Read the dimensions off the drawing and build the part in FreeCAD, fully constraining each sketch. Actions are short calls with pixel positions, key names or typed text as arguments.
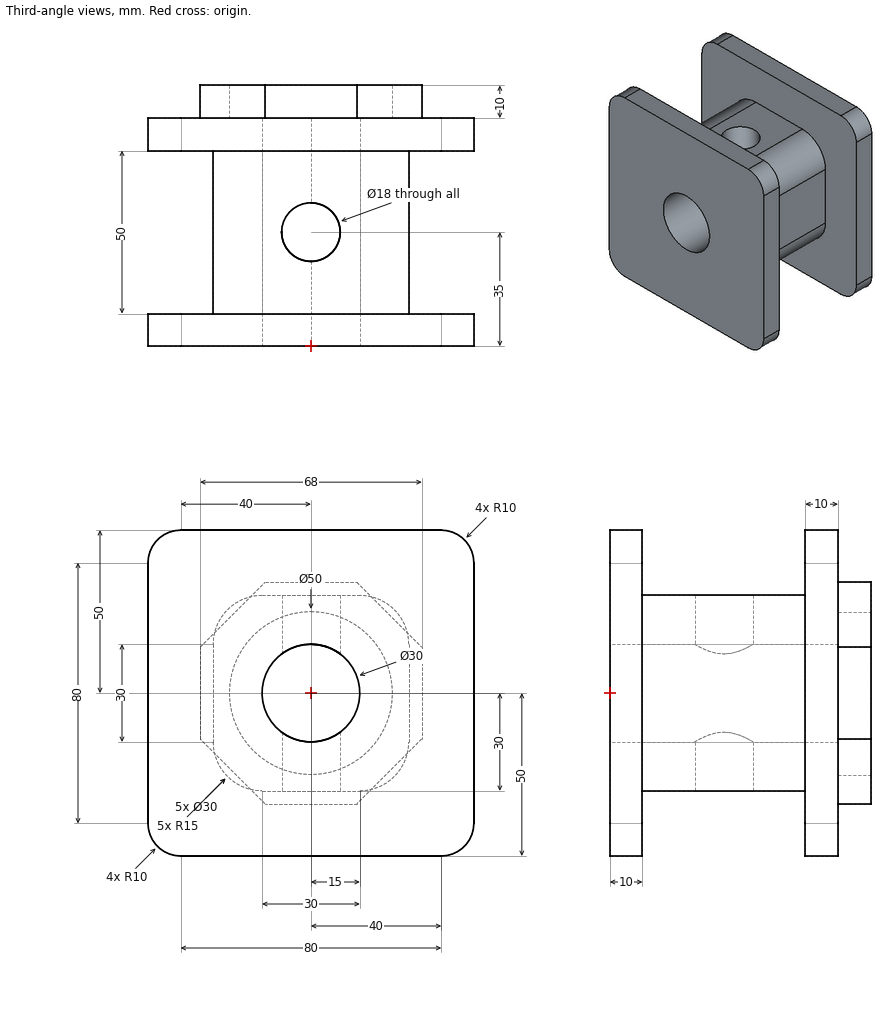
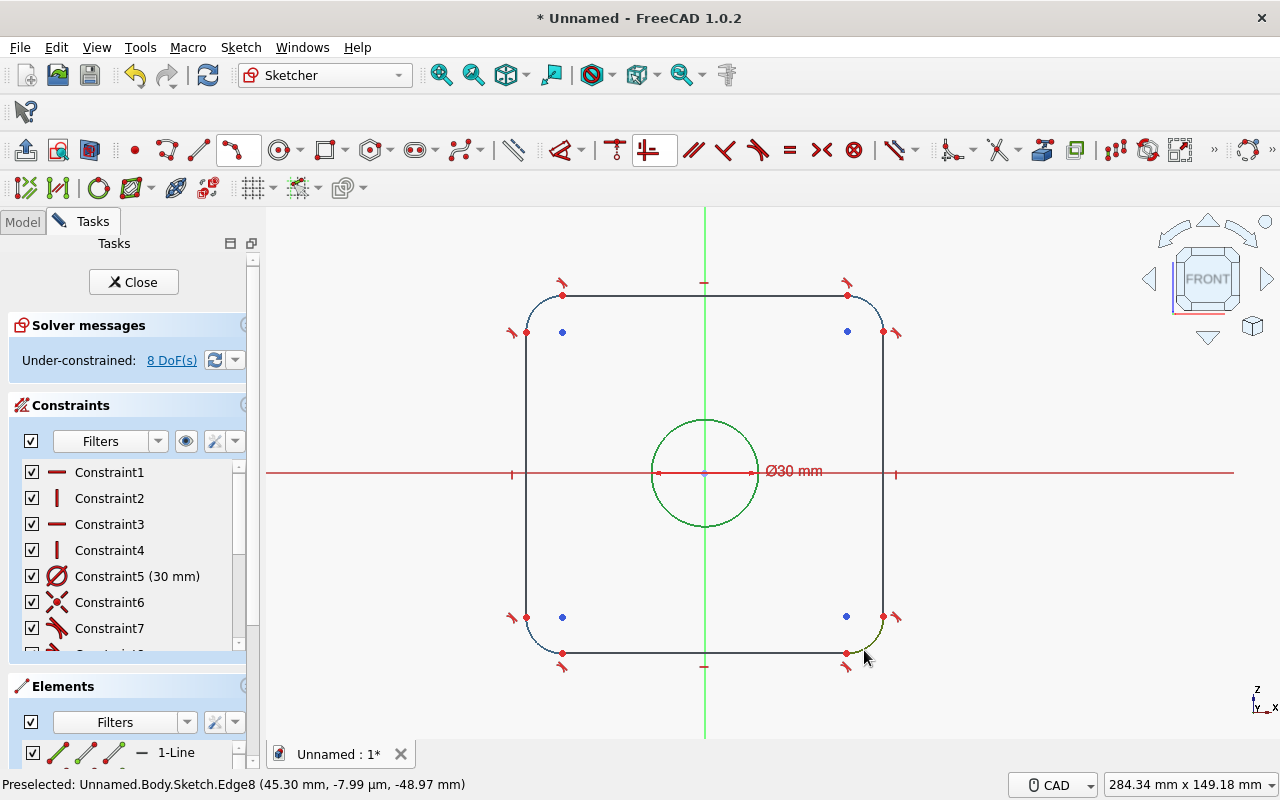
click(790, 150)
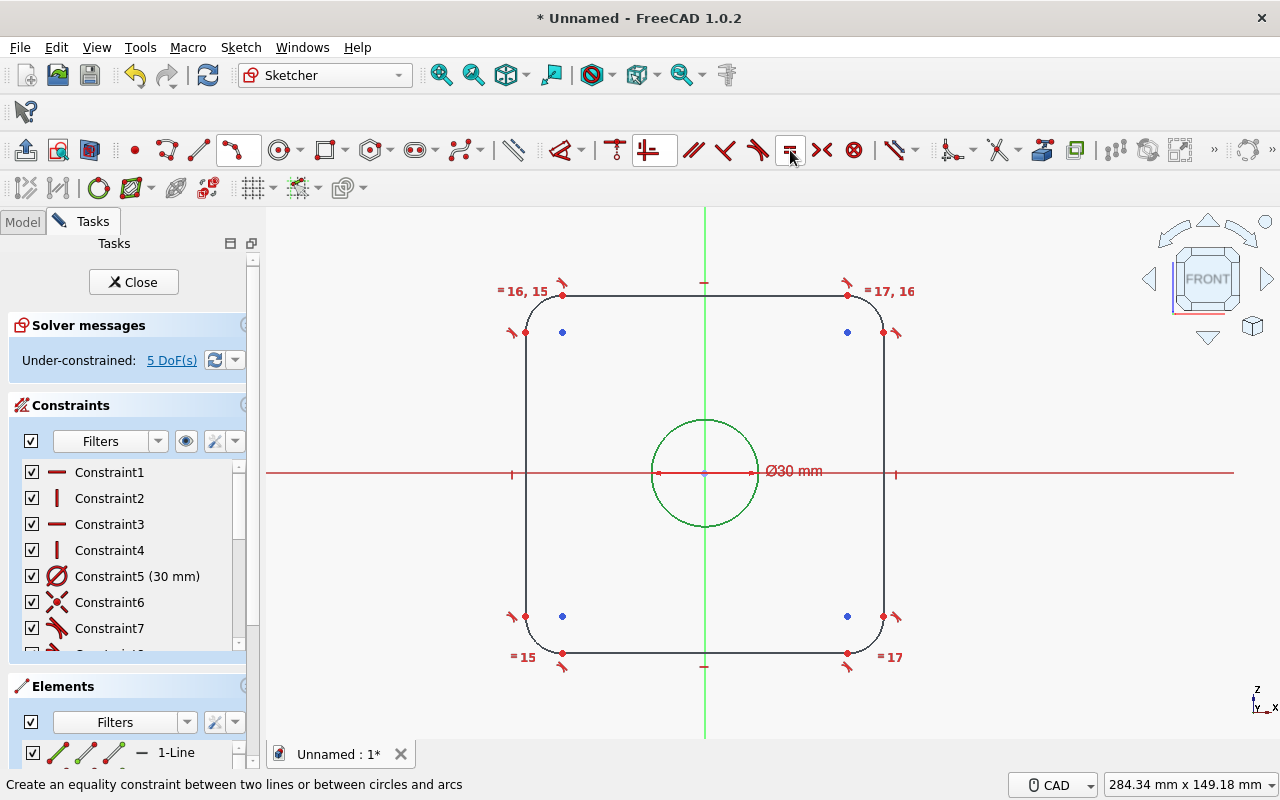
click(560, 150)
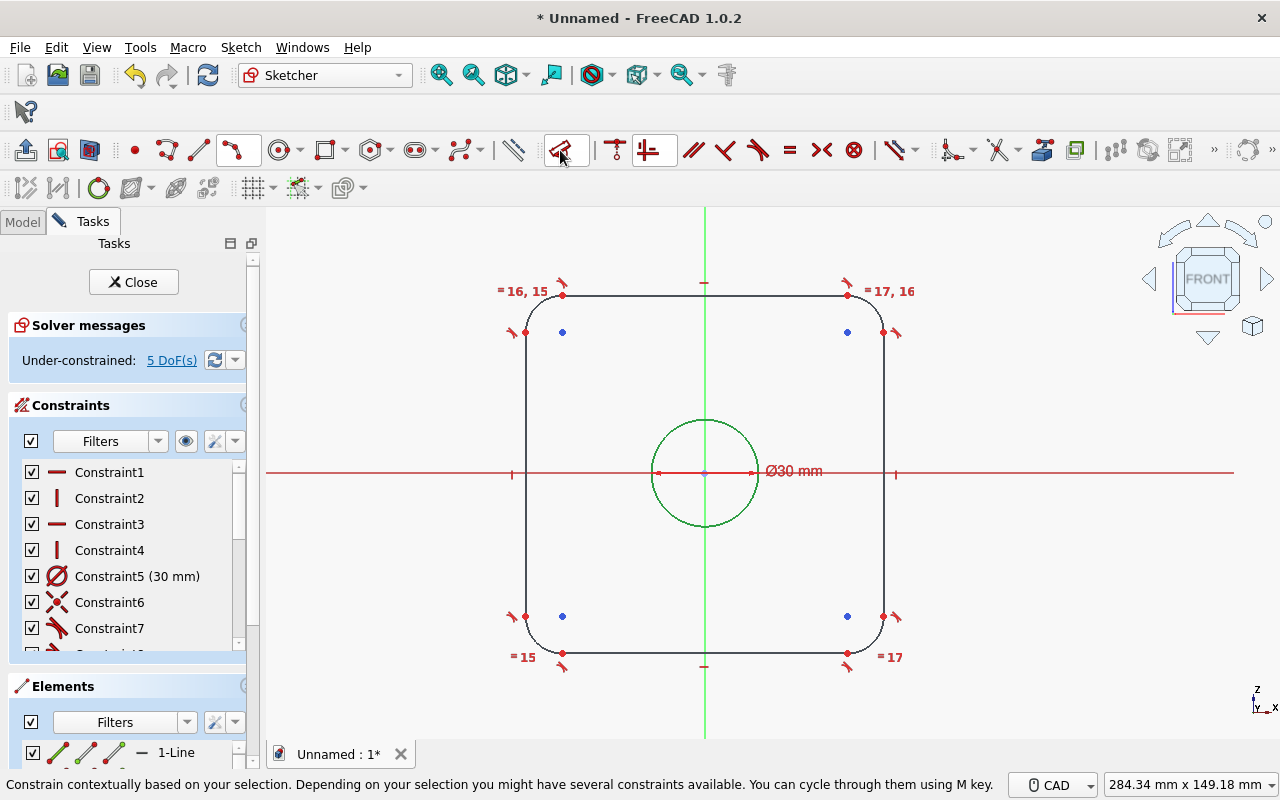
click(530, 634)
click(502, 649)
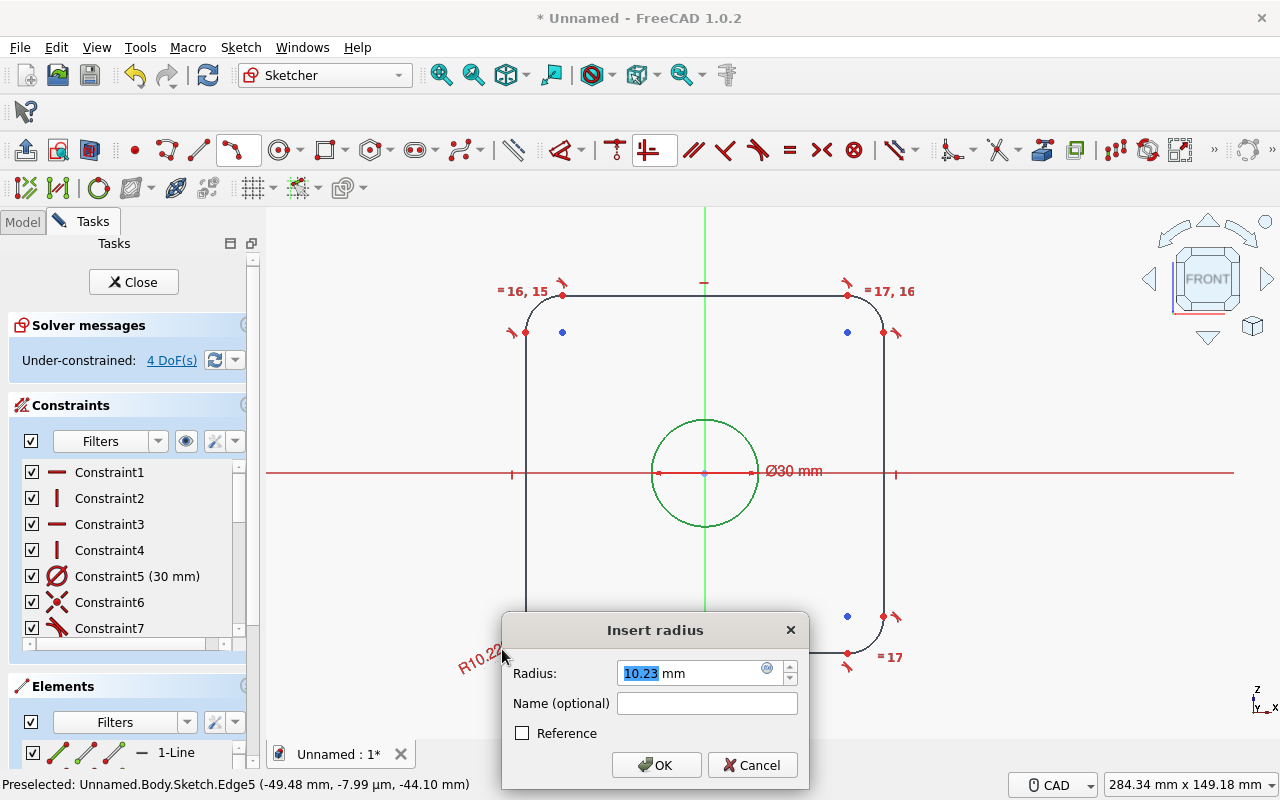
text(10)
key(Return)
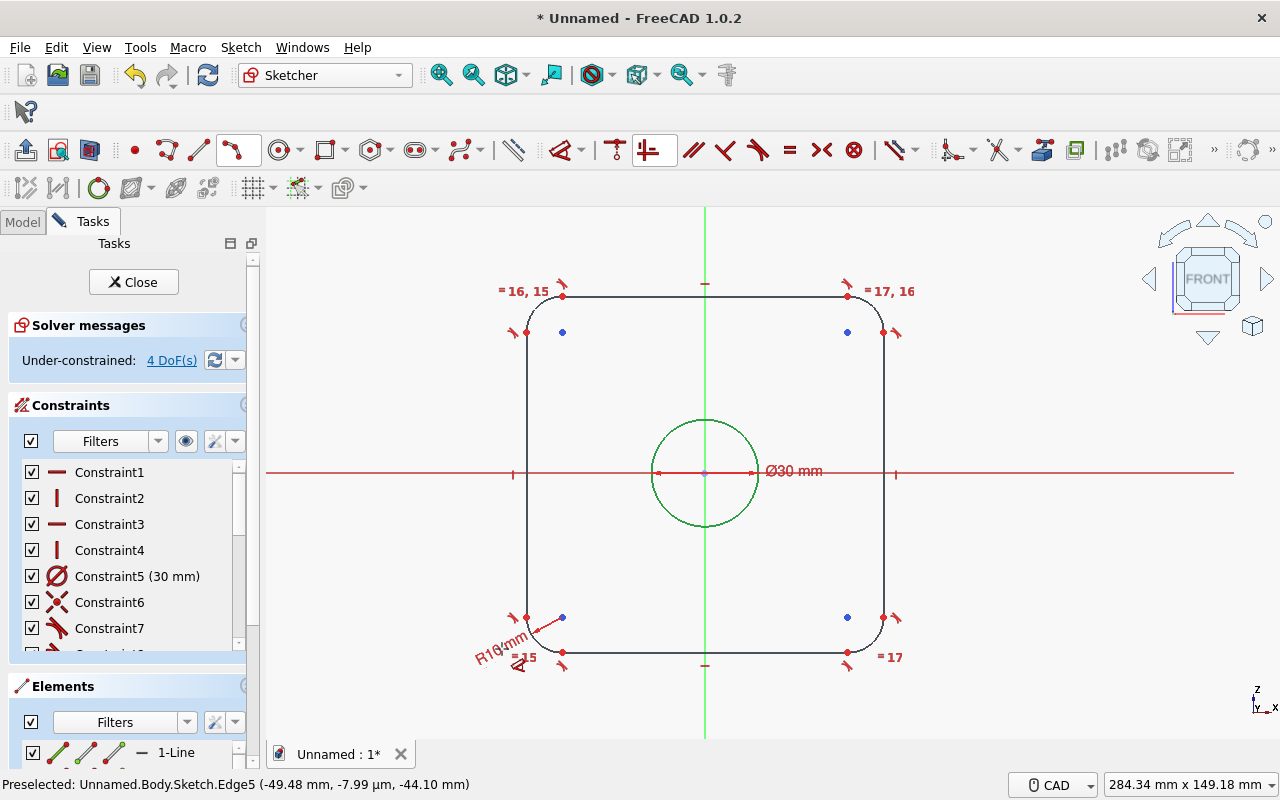
click(762, 653)
click(640, 687)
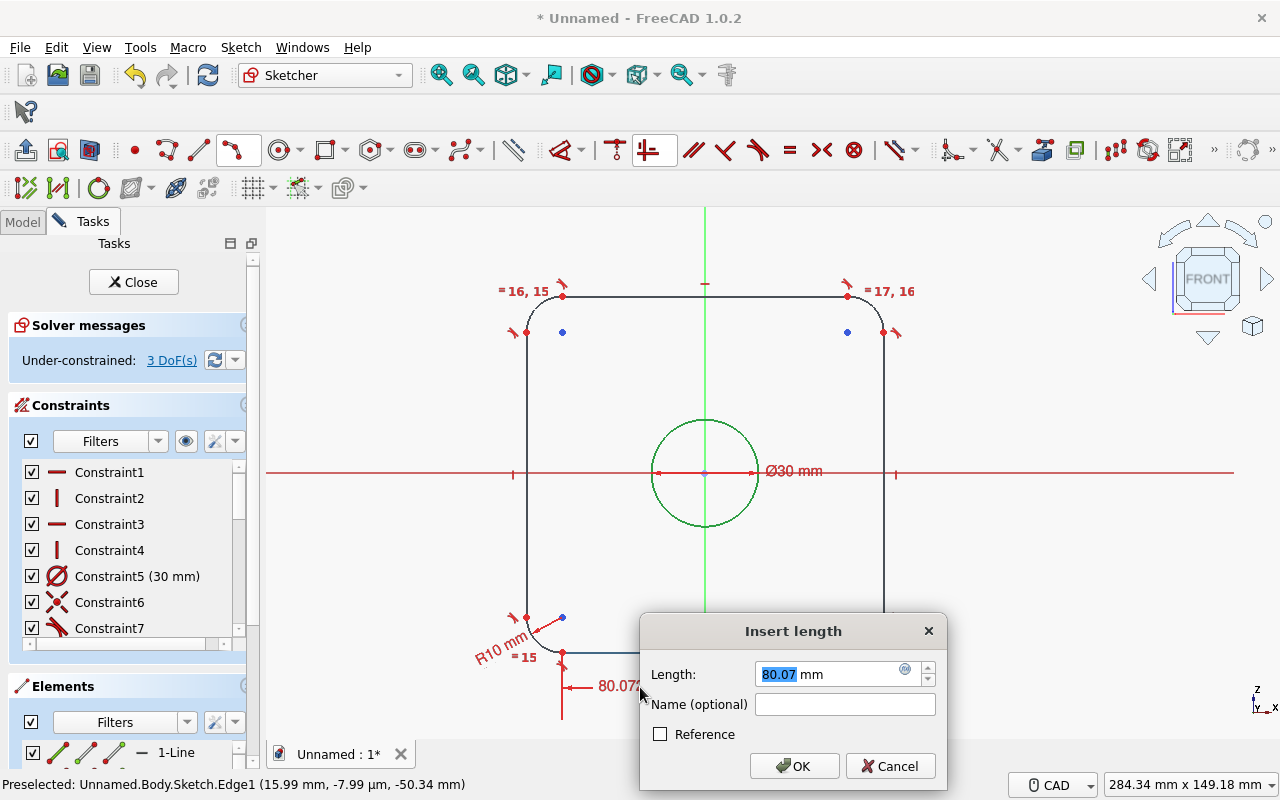
text(80)
key(Return)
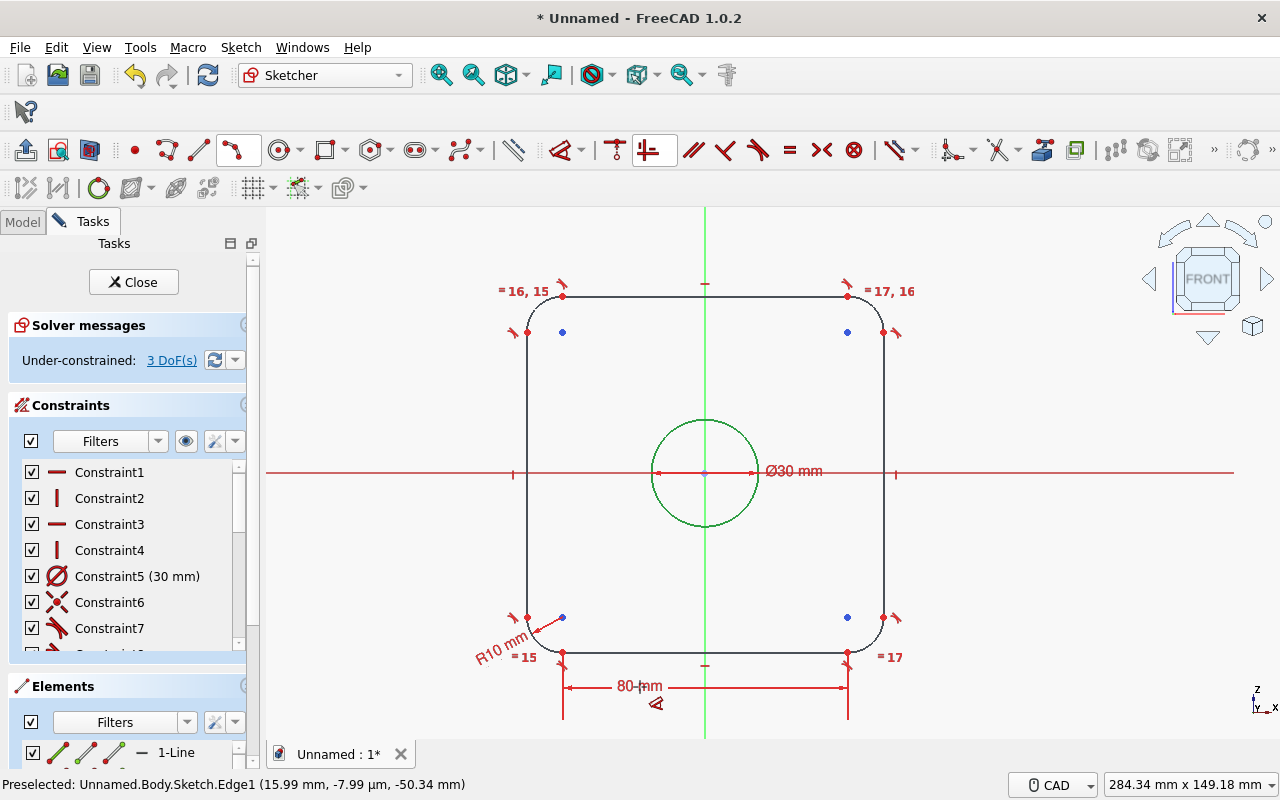
click(527, 532)
click(493, 409)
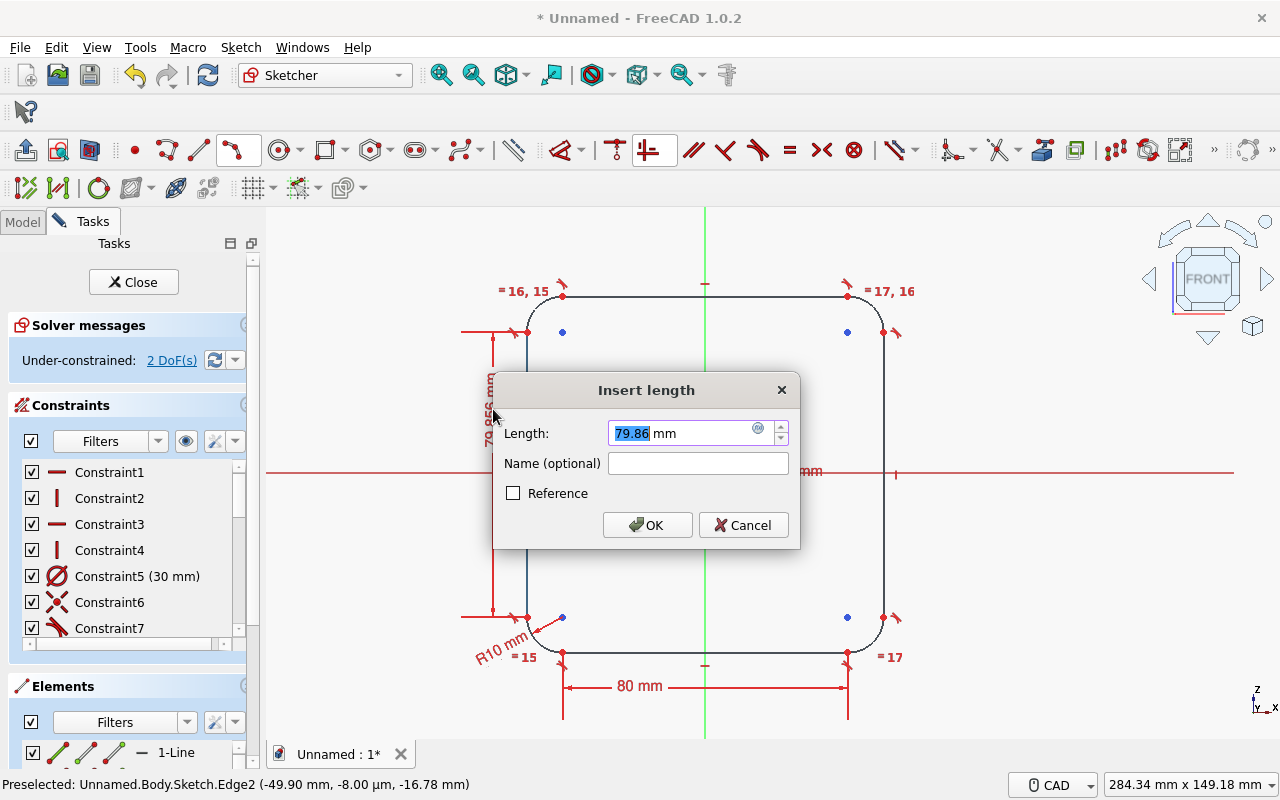
text(80)
key(Return)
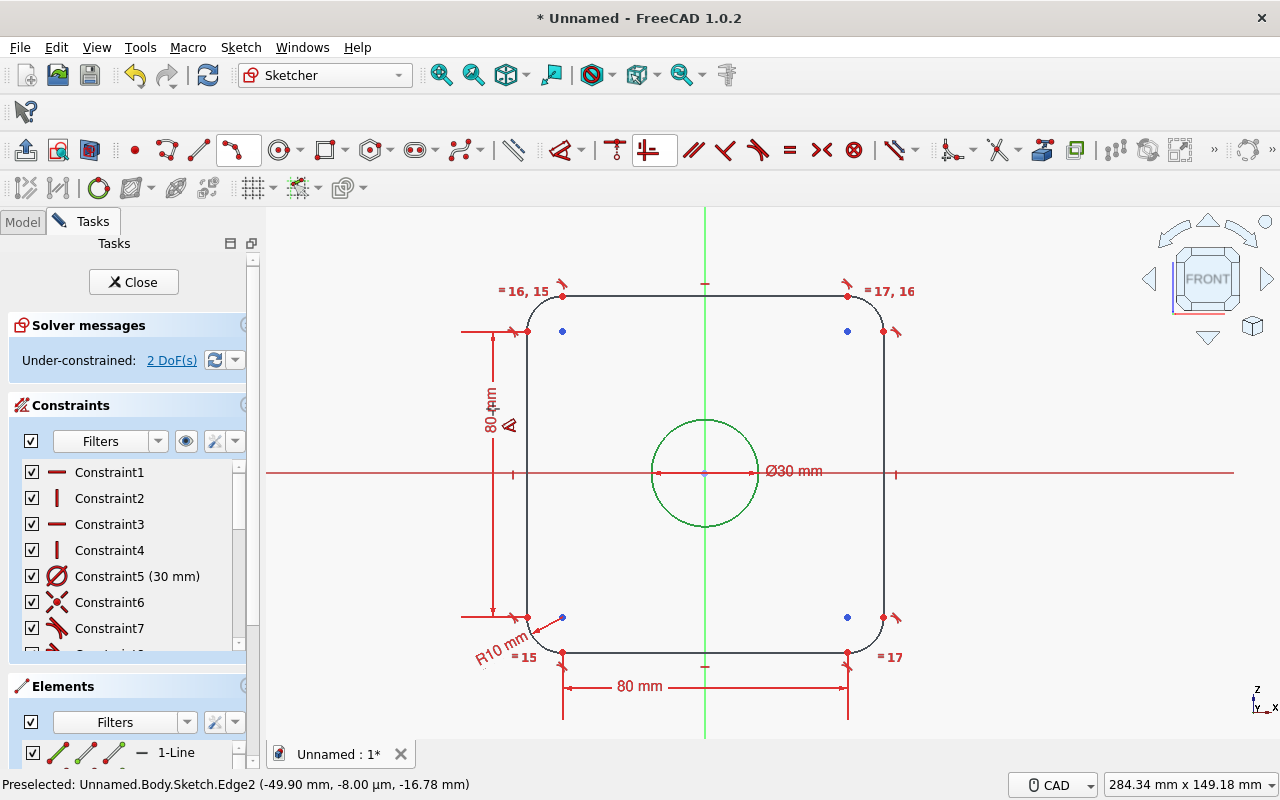
click(848, 653)
click(776, 687)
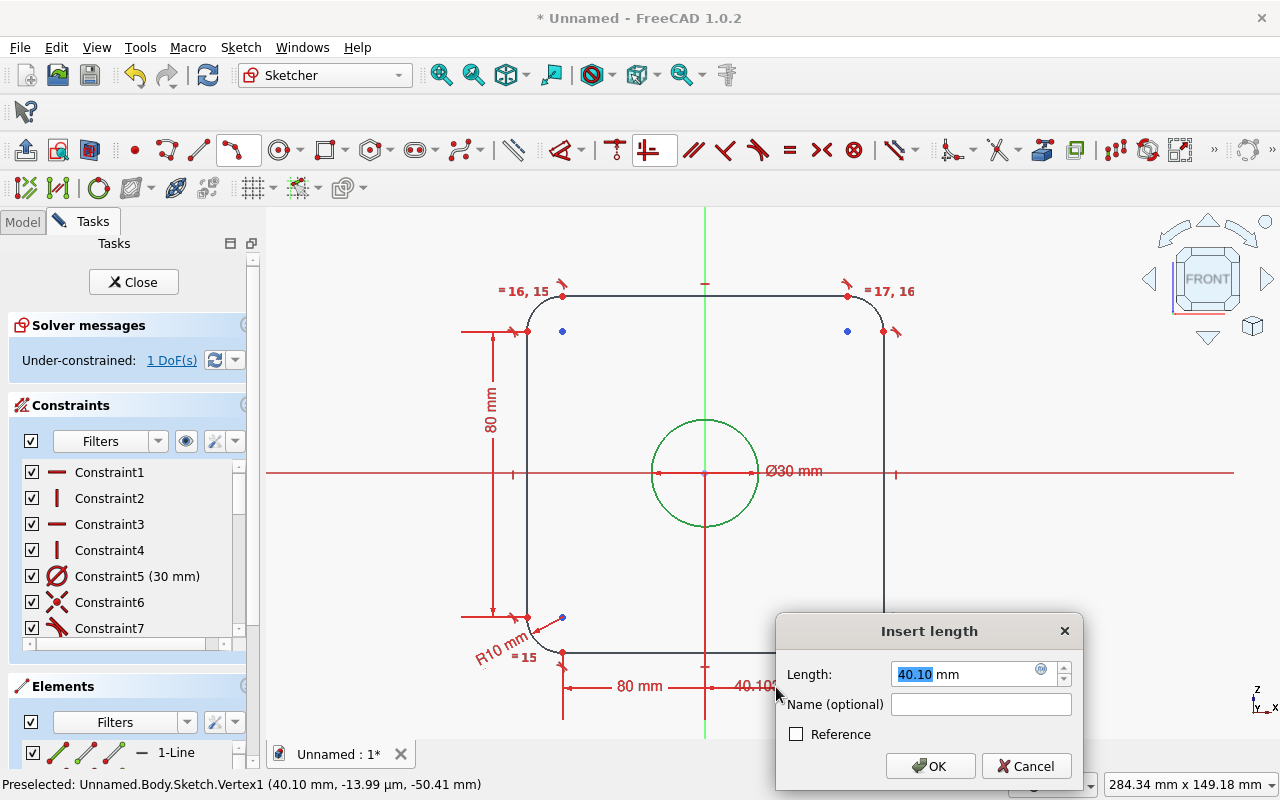
text(40)
key(Return)